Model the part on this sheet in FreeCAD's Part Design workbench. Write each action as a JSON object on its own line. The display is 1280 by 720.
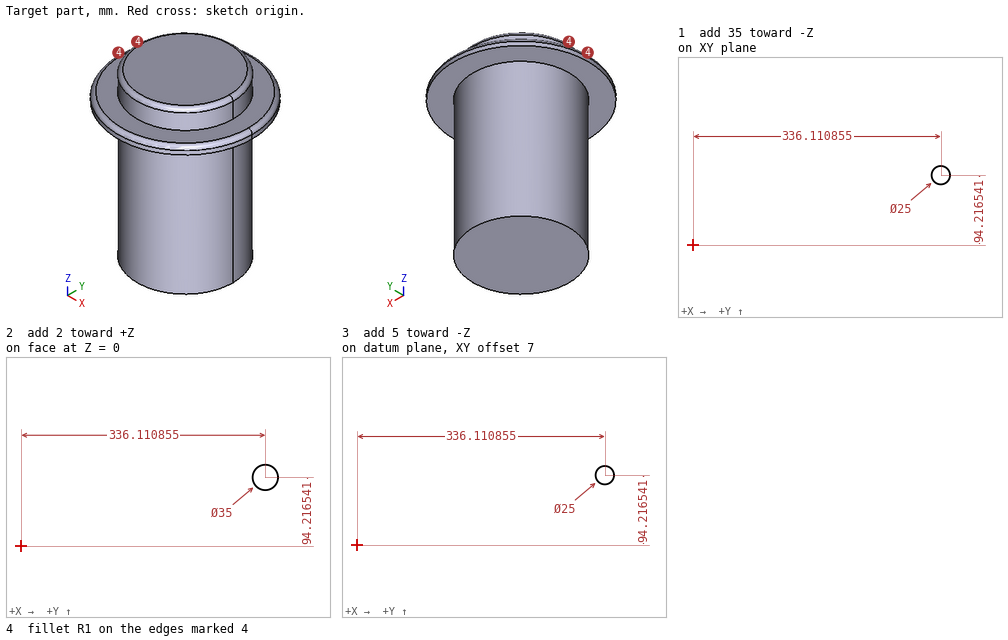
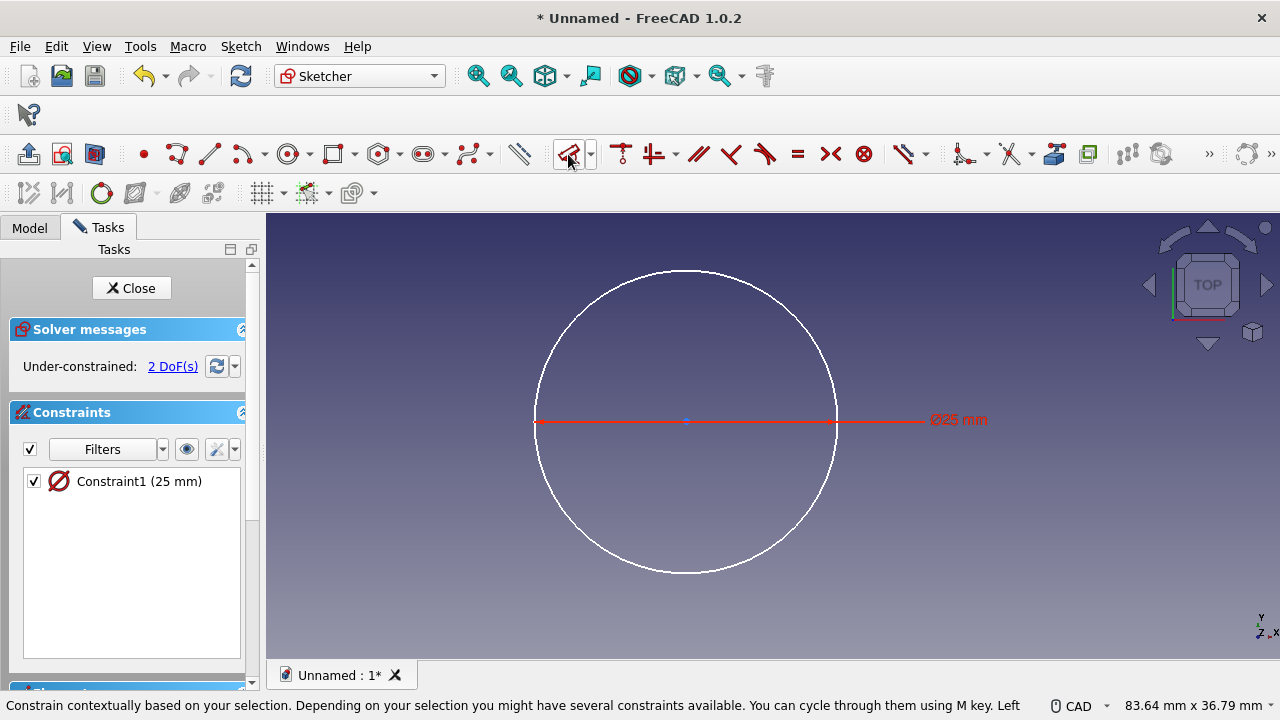
{"action": "left_click", "coordinate": [686, 422]}
{"action": "left_click", "coordinate": [720, 527]}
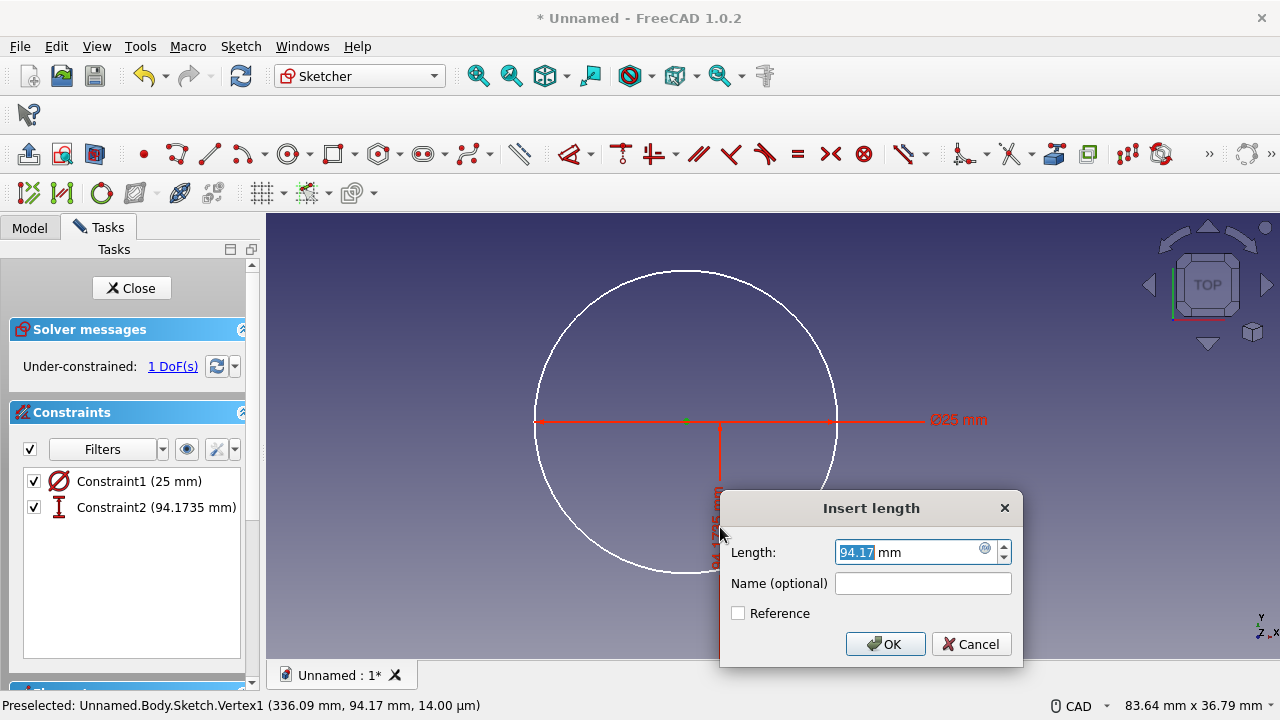
{"action": "type", "text": "94.216541"}
{"action": "key", "text": "Return"}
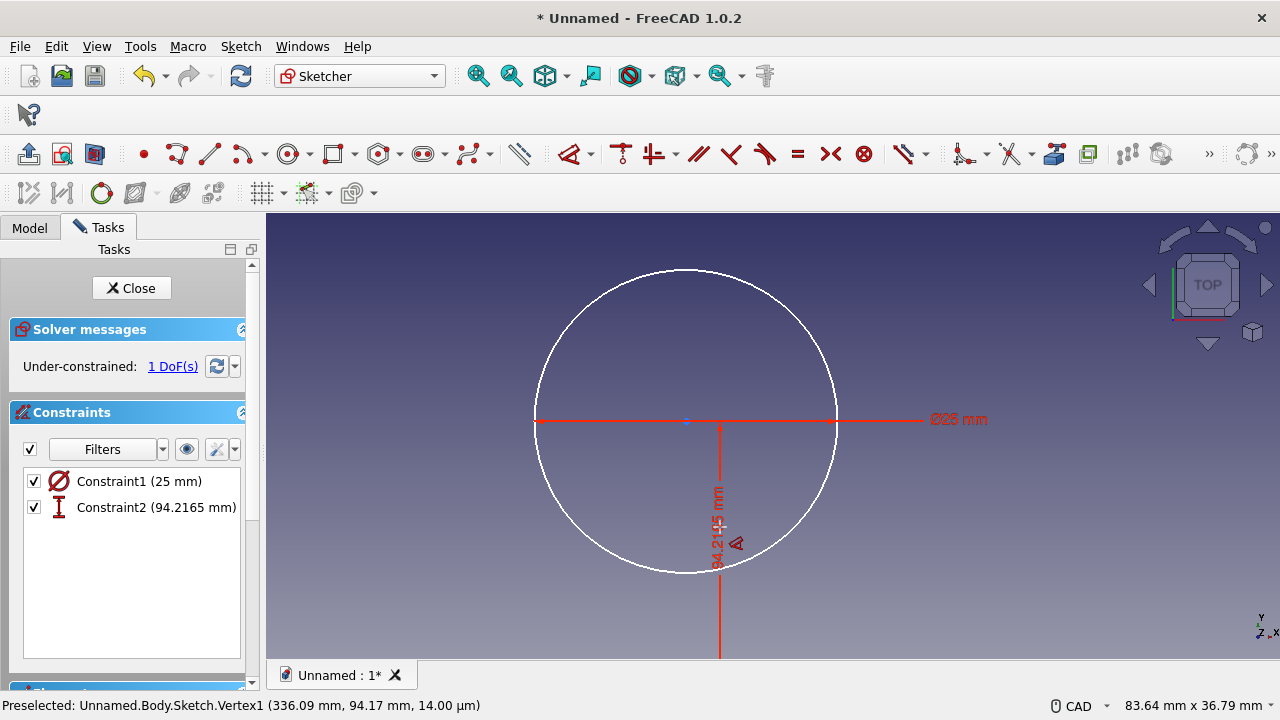
{"action": "left_click", "coordinate": [686, 421]}
{"action": "left_click", "coordinate": [490, 387]}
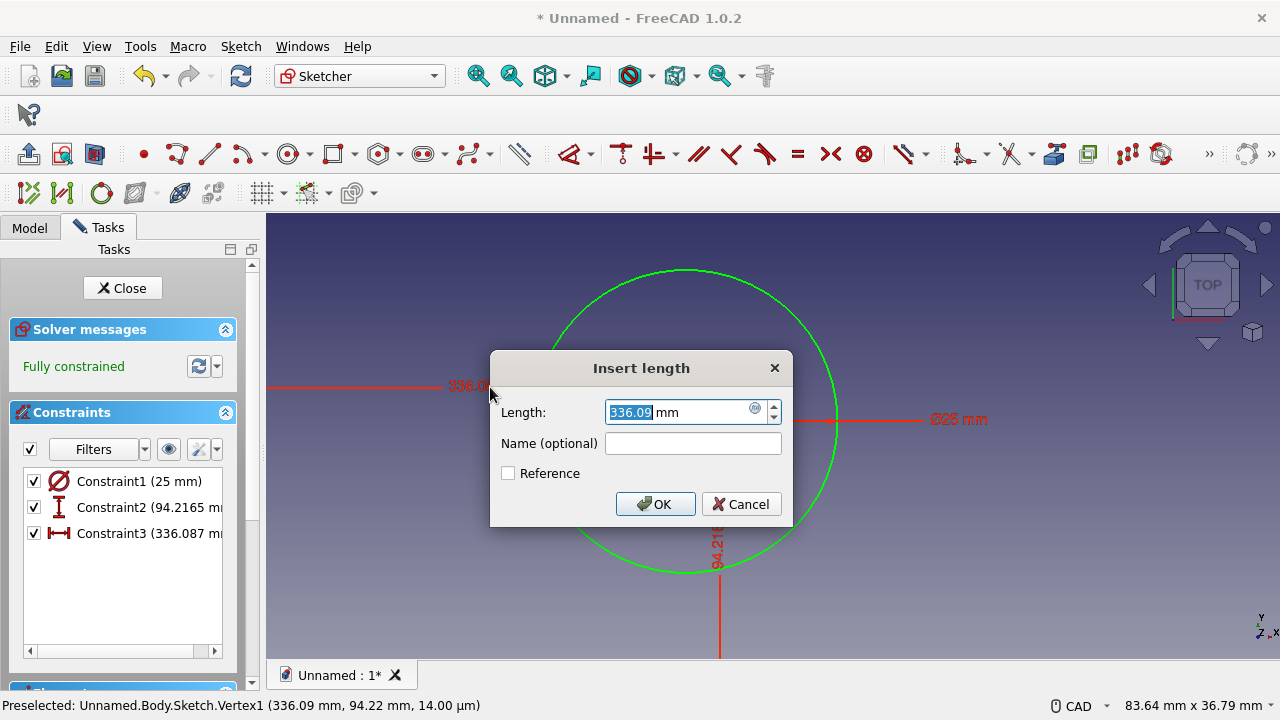
{"action": "type", "text": "336.110855"}
{"action": "key", "text": "Return"}
{"action": "key", "text": "Escape"}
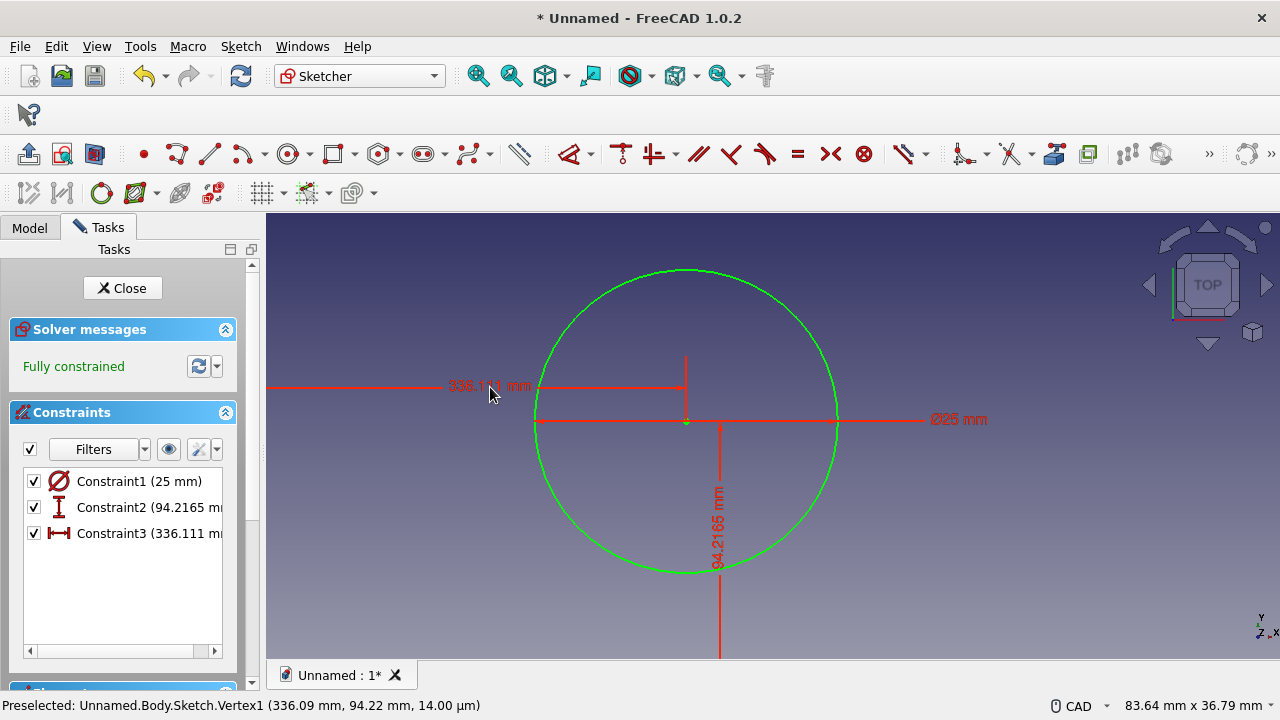
{"action": "left_click", "coordinate": [123, 288]}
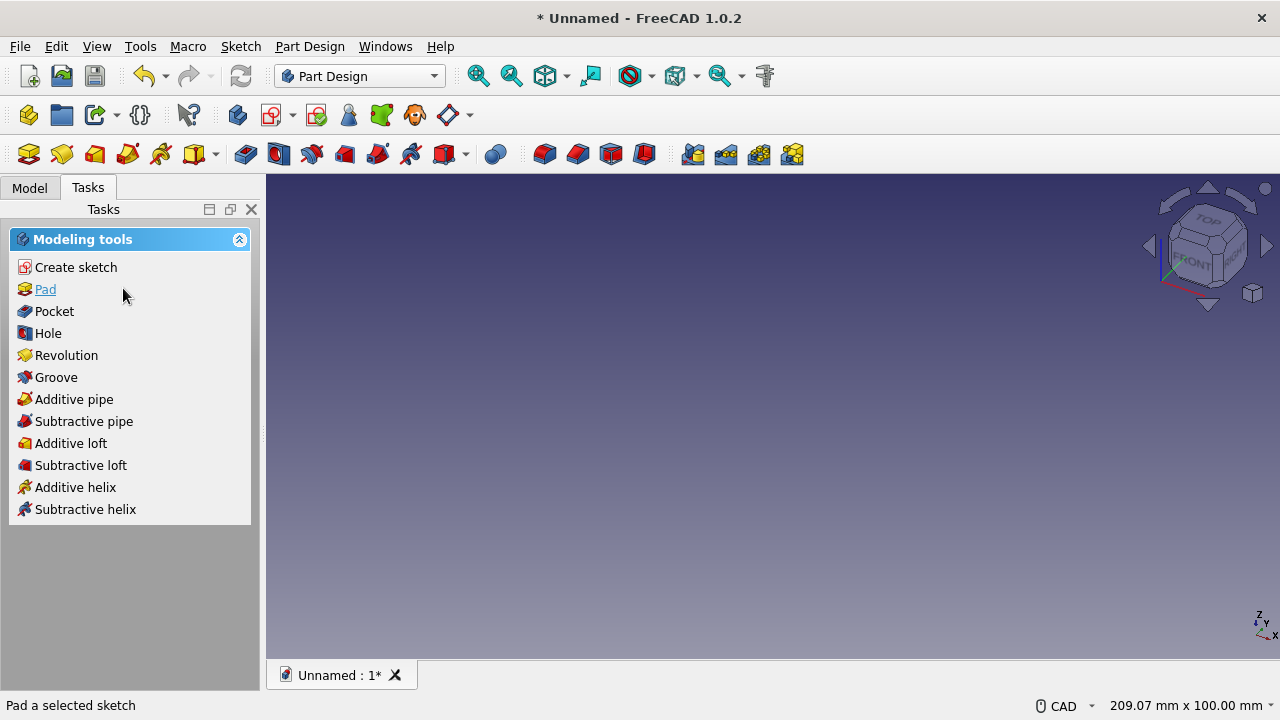
{"action": "left_click", "coordinate": [29, 154]}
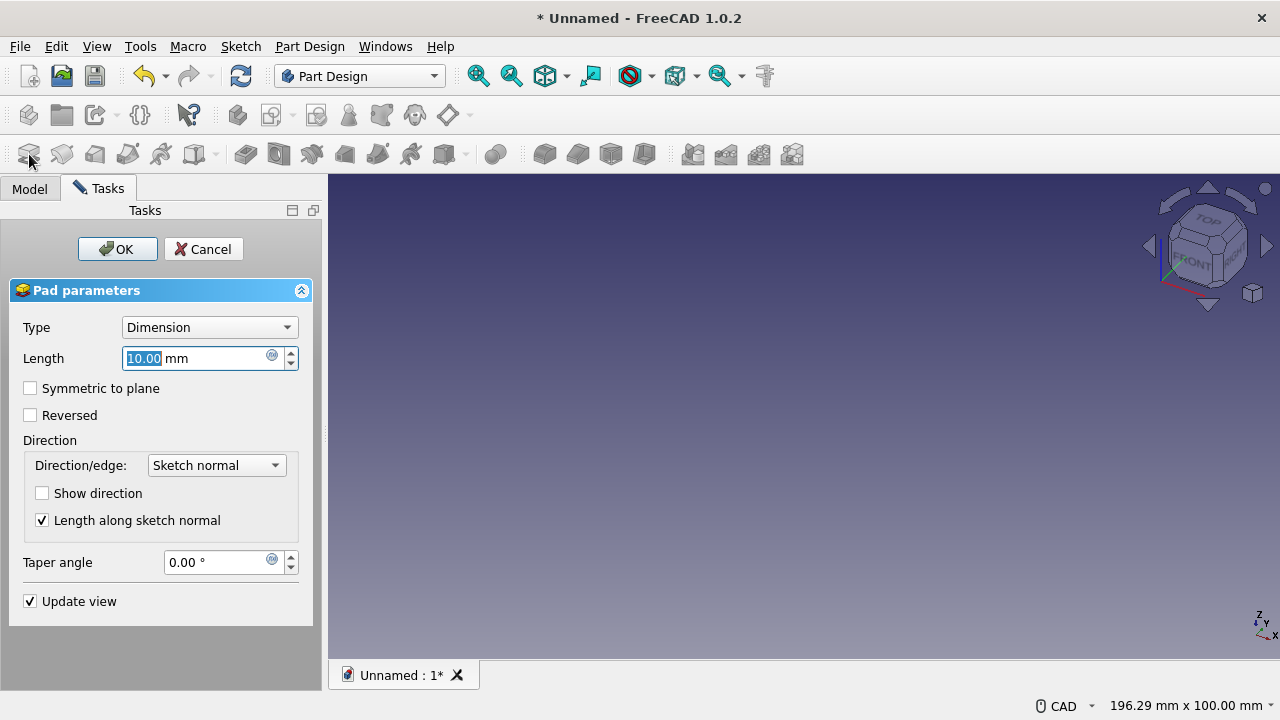
{"action": "type", "text": "35"}
{"action": "key", "text": "Tab"}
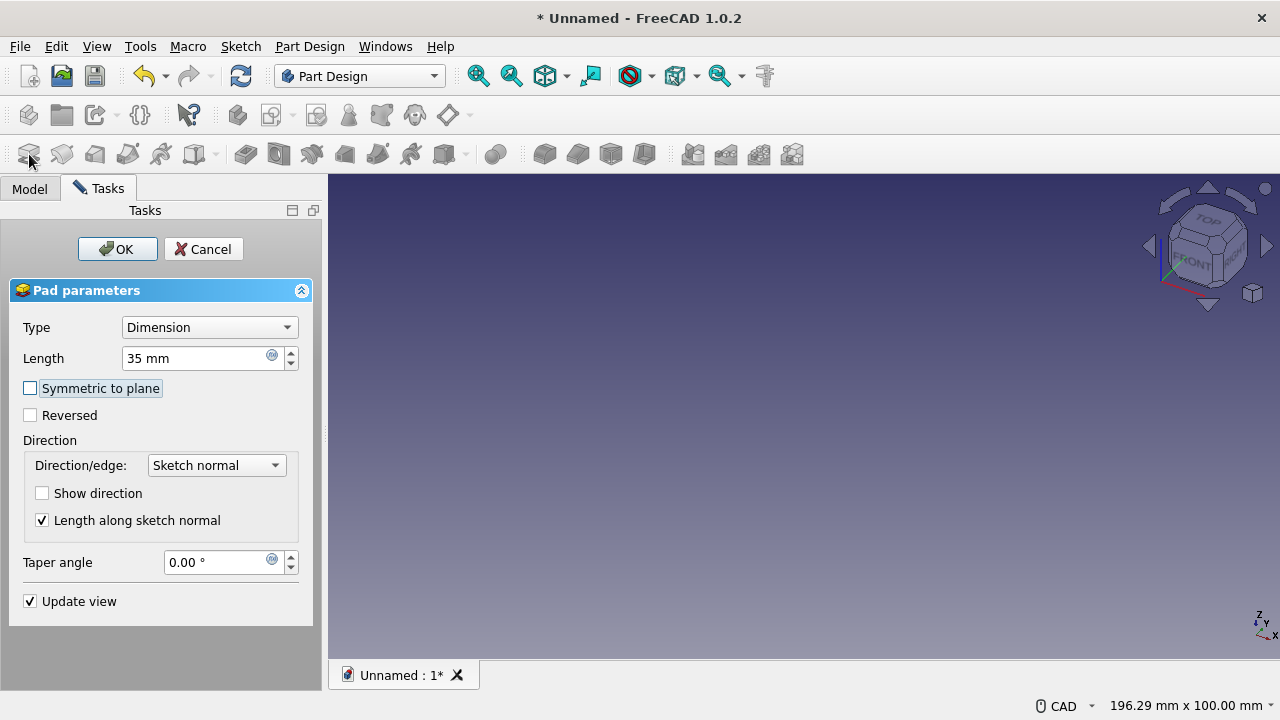
{"action": "left_click", "coordinate": [31, 415]}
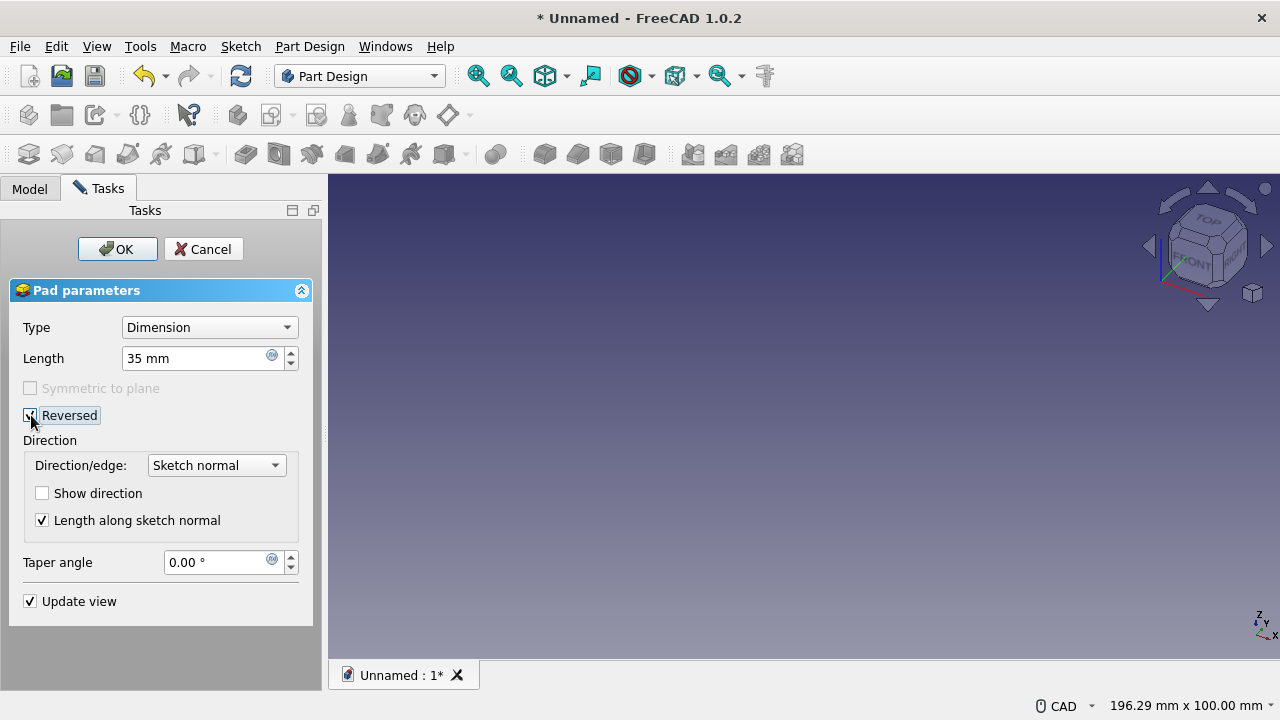
{"action": "left_click", "coordinate": [118, 249]}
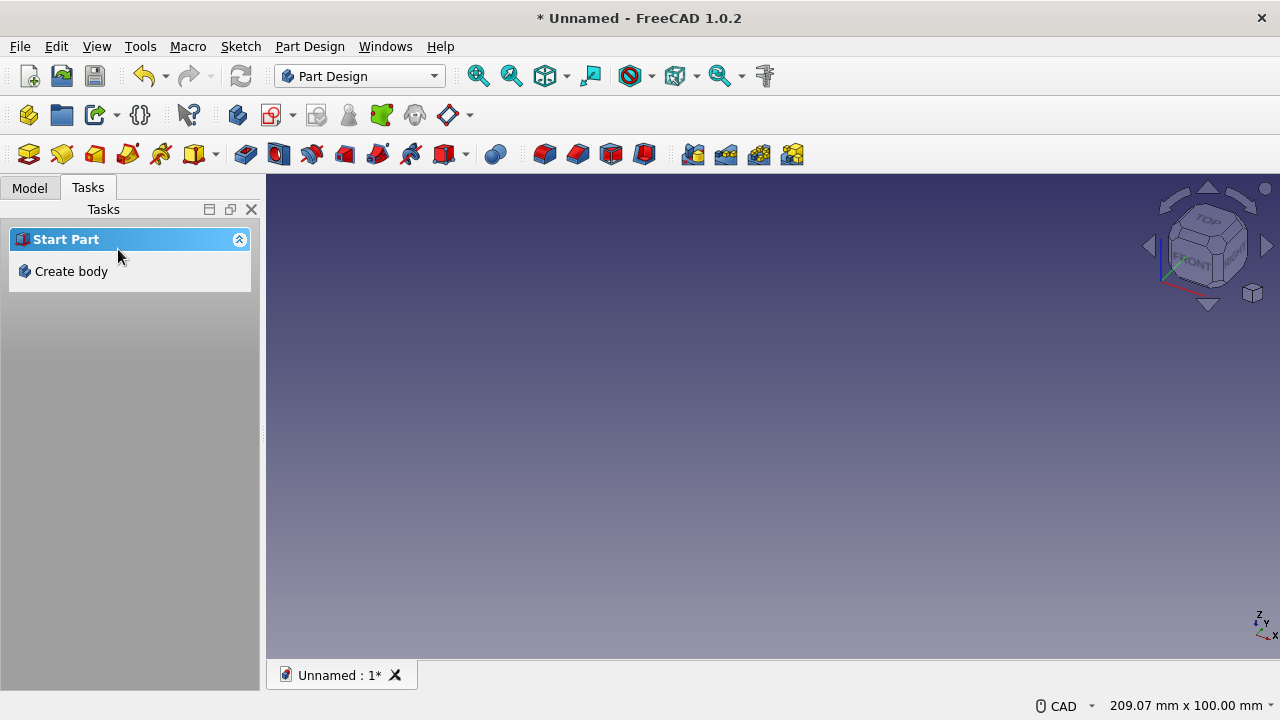
{"action": "left_click", "coordinate": [479, 76]}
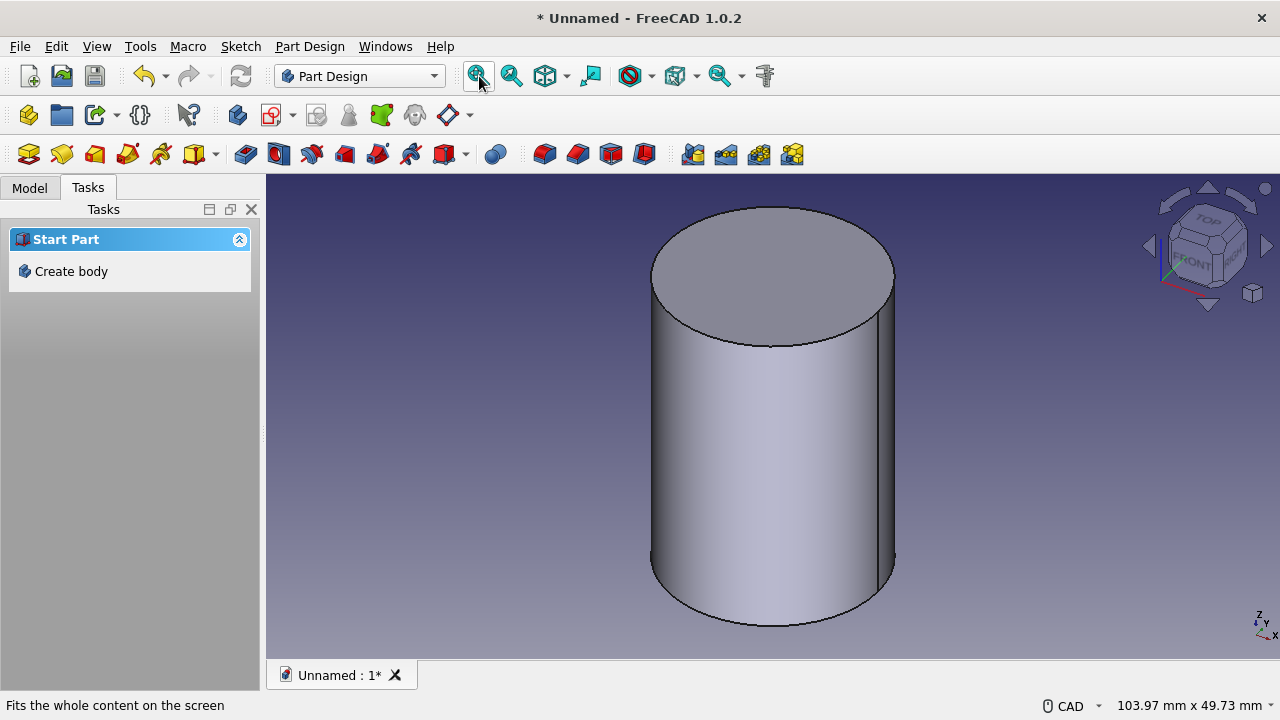
{"action": "left_click", "coordinate": [773, 276]}